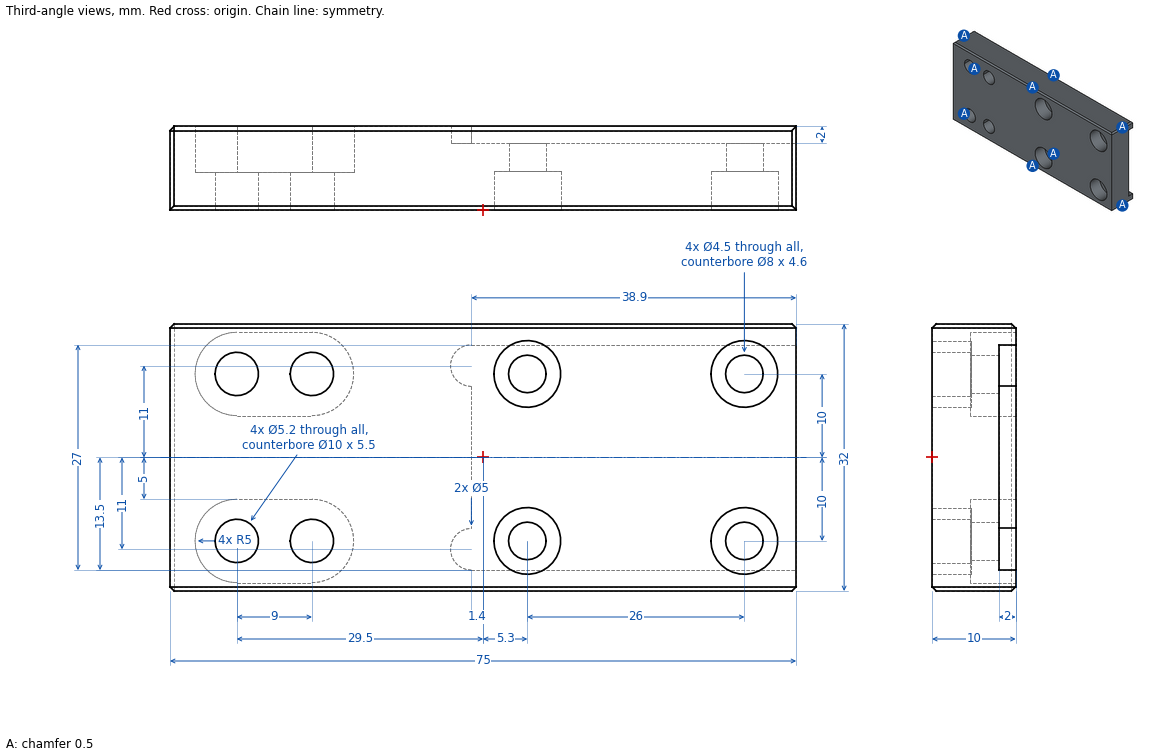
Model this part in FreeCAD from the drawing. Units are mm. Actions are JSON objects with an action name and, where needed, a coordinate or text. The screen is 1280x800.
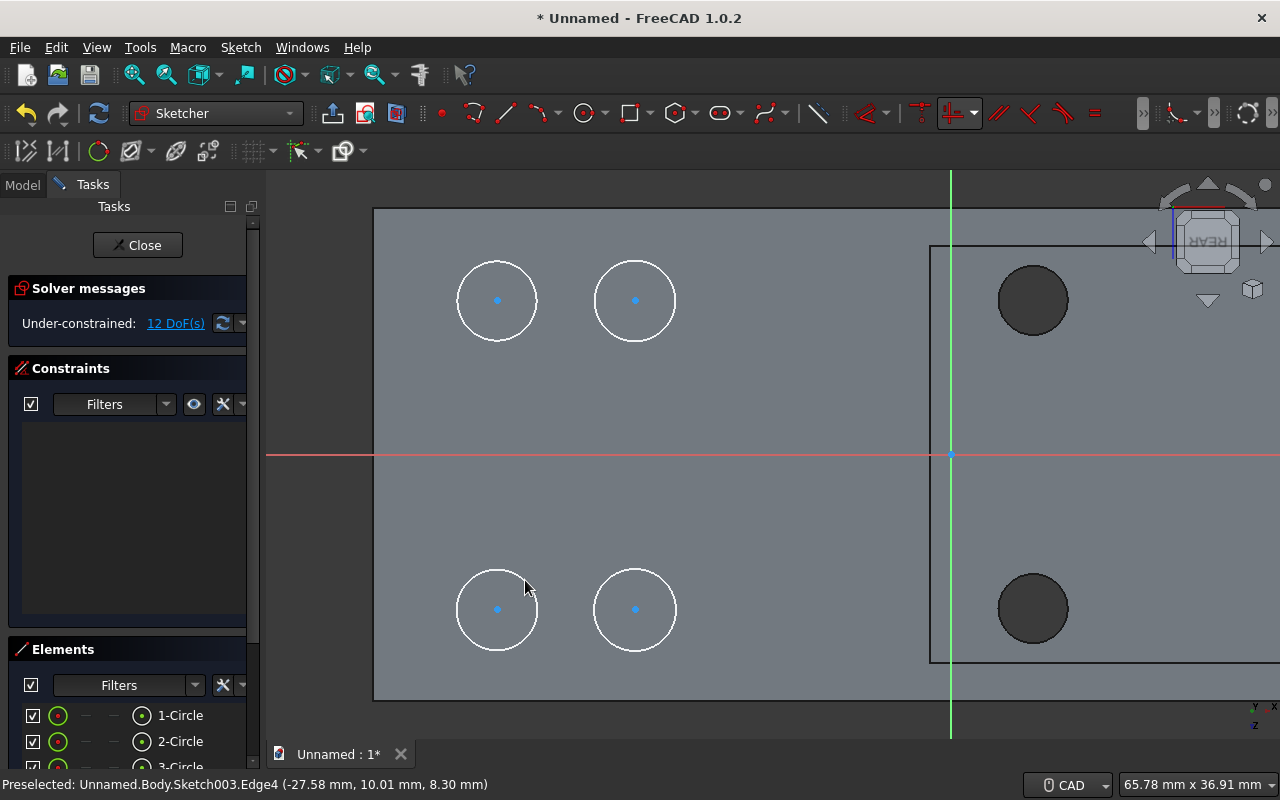
{"action": "left_click", "coordinate": [525, 273]}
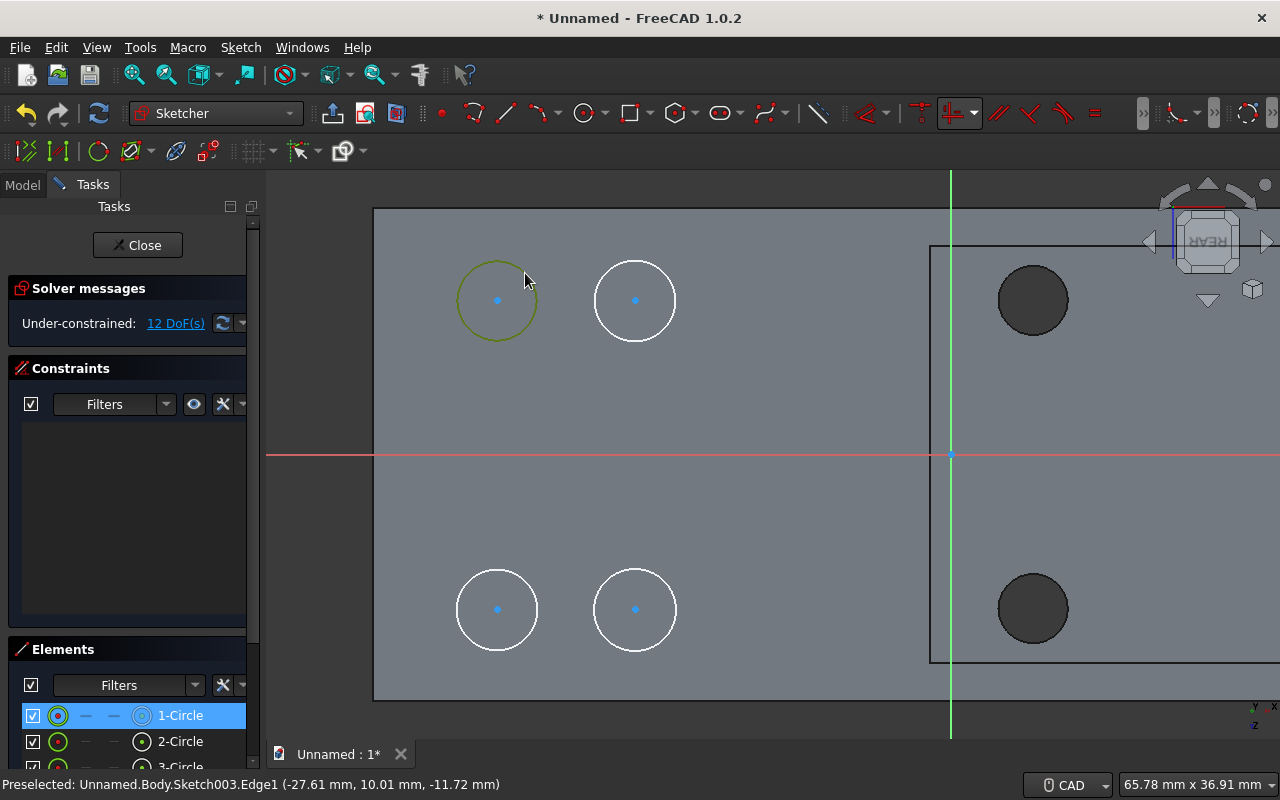
{"action": "left_click", "coordinate": [663, 272]}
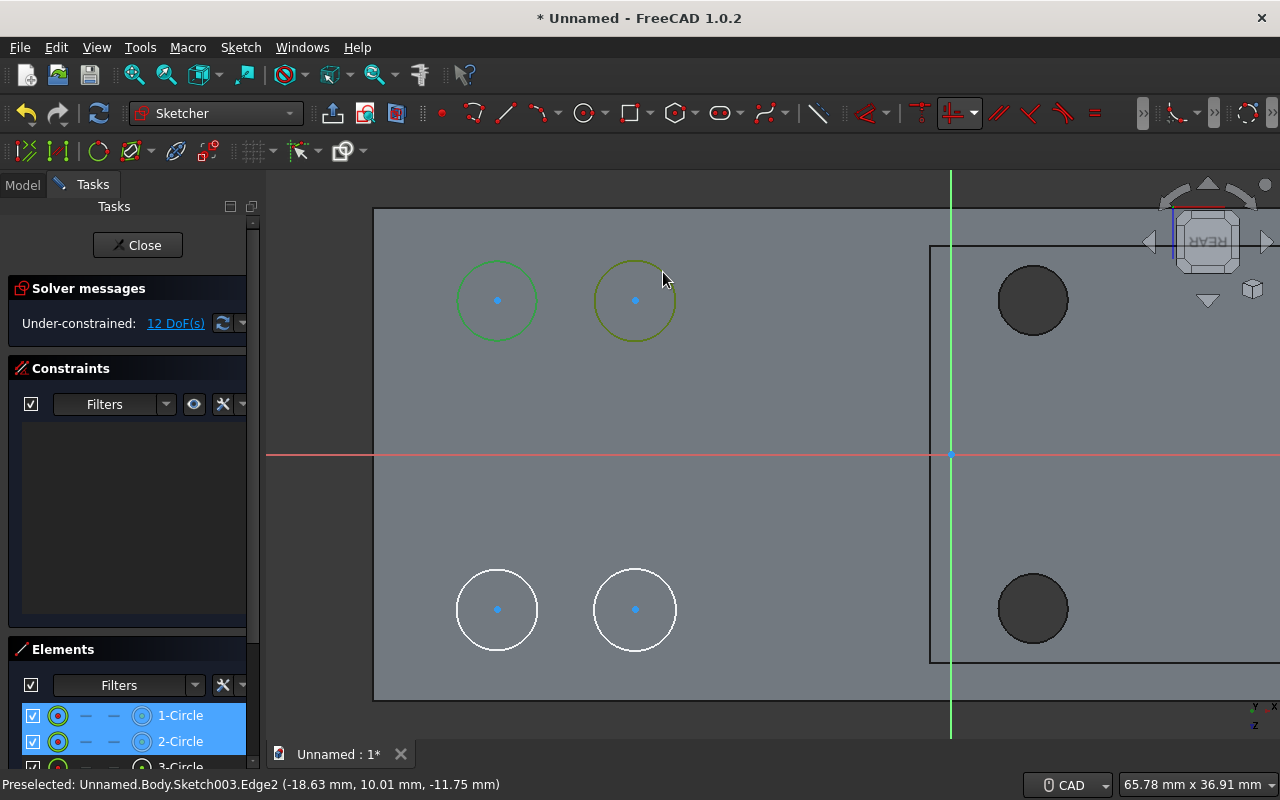
{"action": "left_click", "coordinate": [664, 581]}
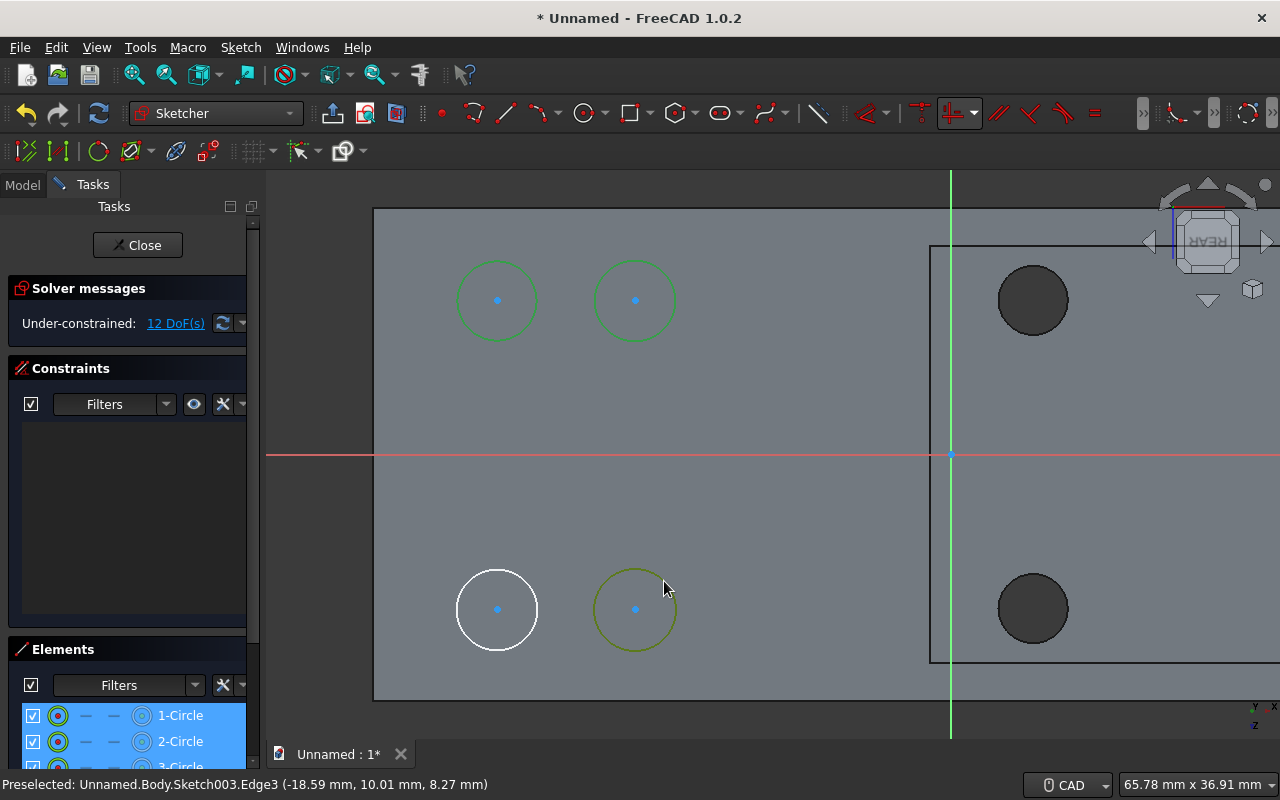
{"action": "left_click", "coordinate": [525, 581]}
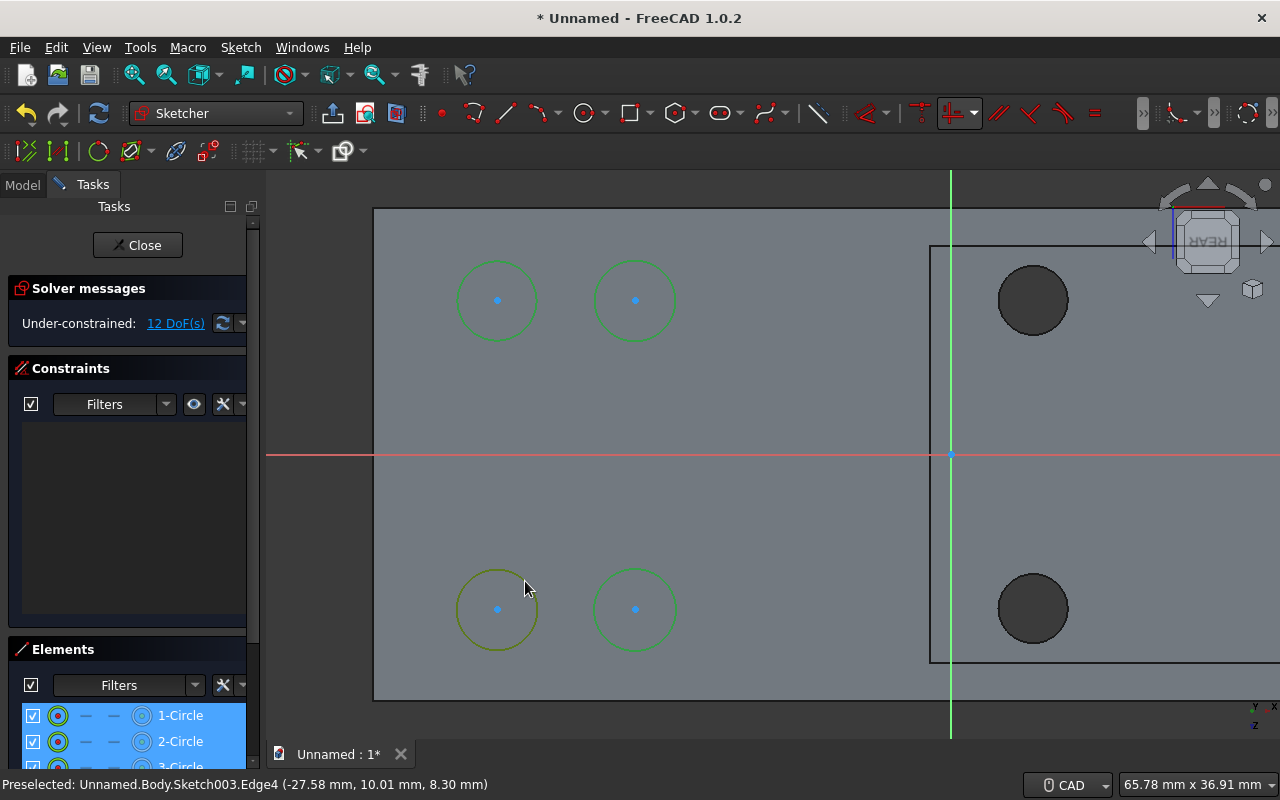
{"action": "left_click", "coordinate": [1096, 114]}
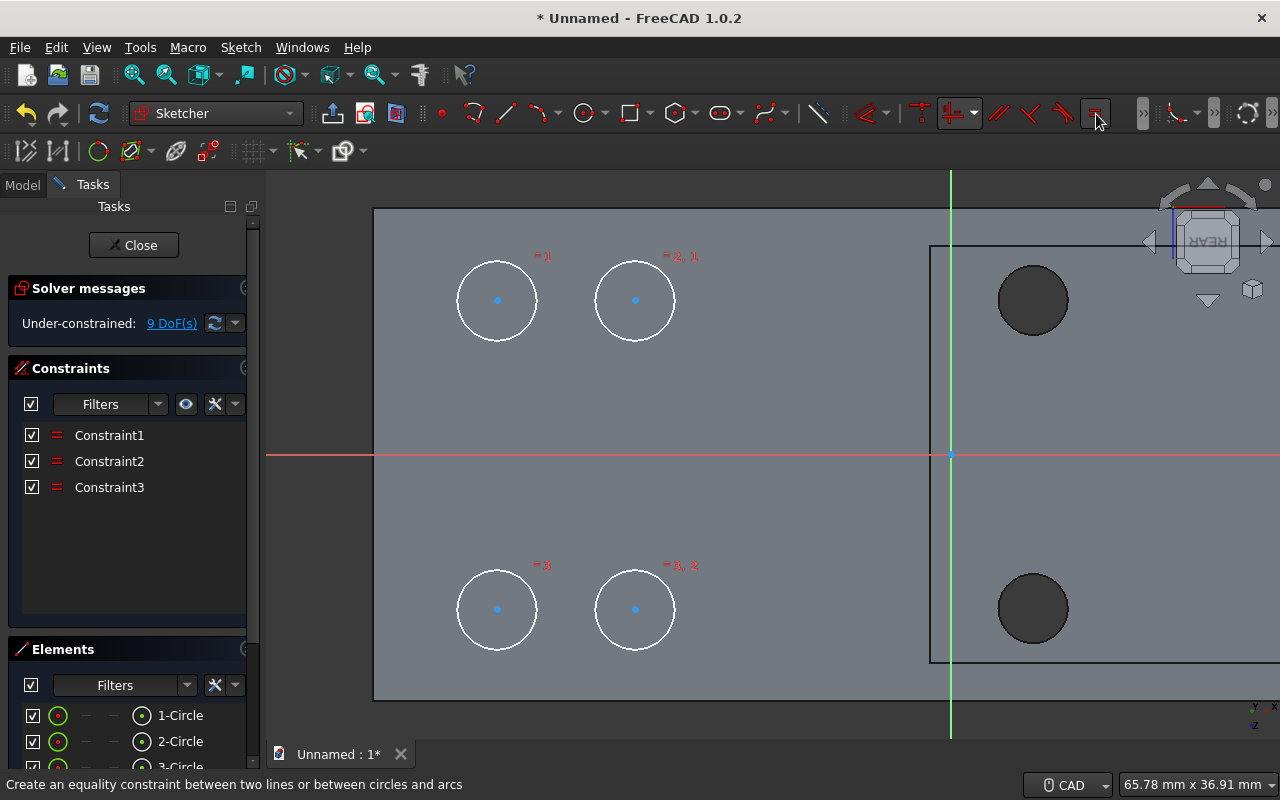
{"action": "left_click", "coordinate": [497, 301]}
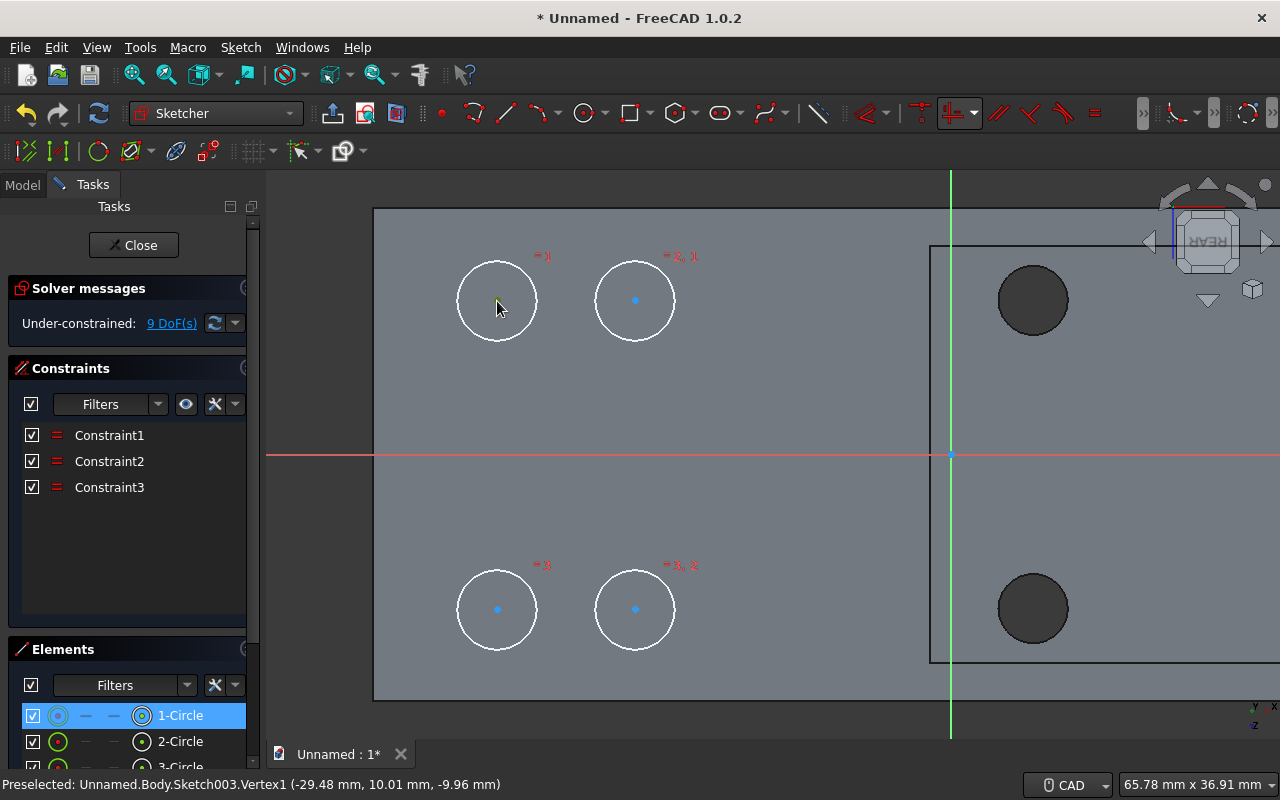
{"action": "left_click", "coordinate": [635, 301]}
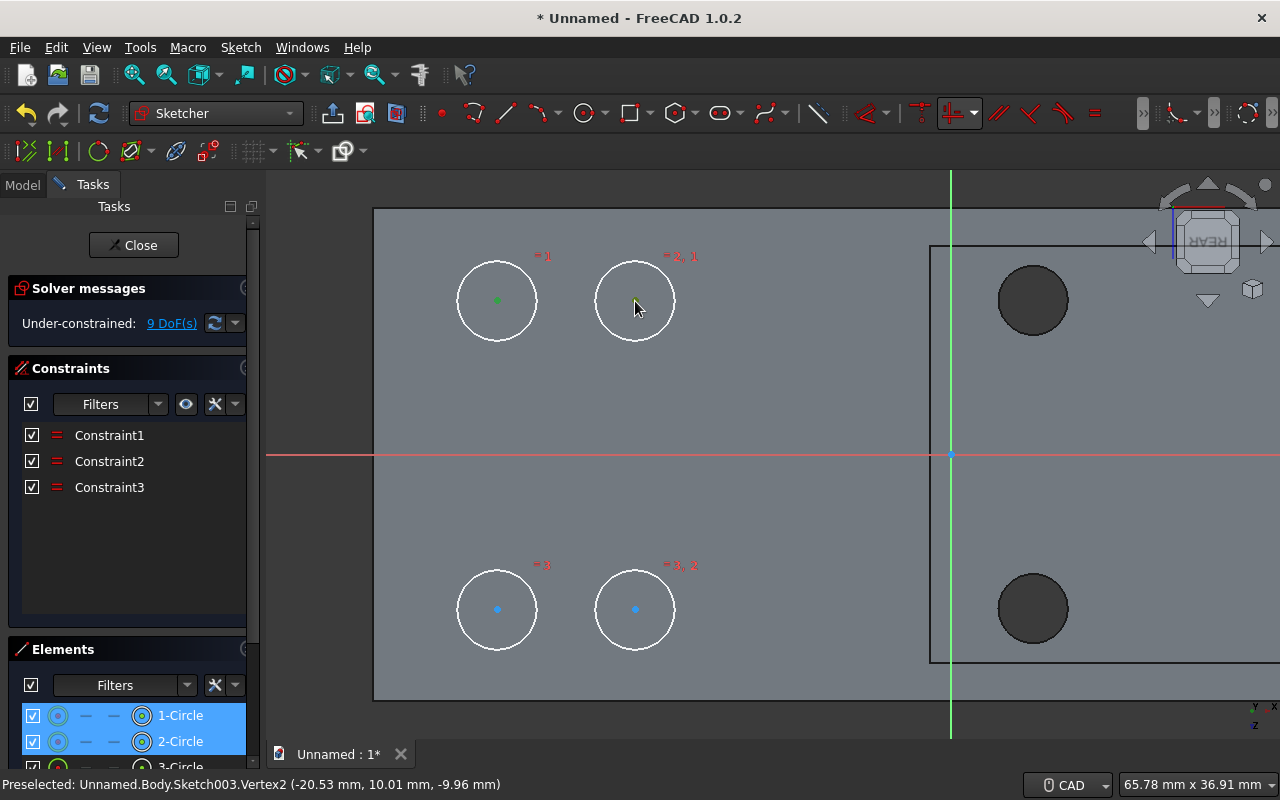
{"action": "left_click", "coordinate": [976, 114]}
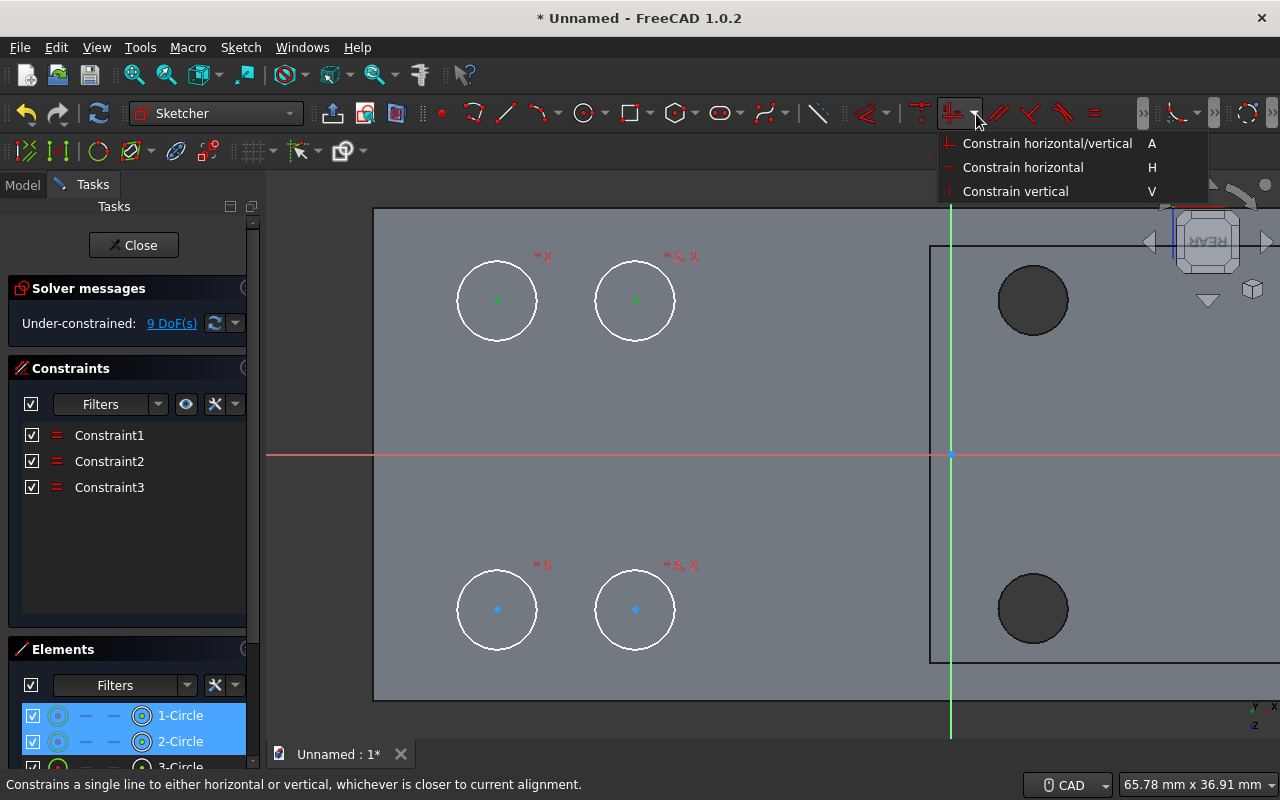
{"action": "left_click", "coordinate": [1073, 167]}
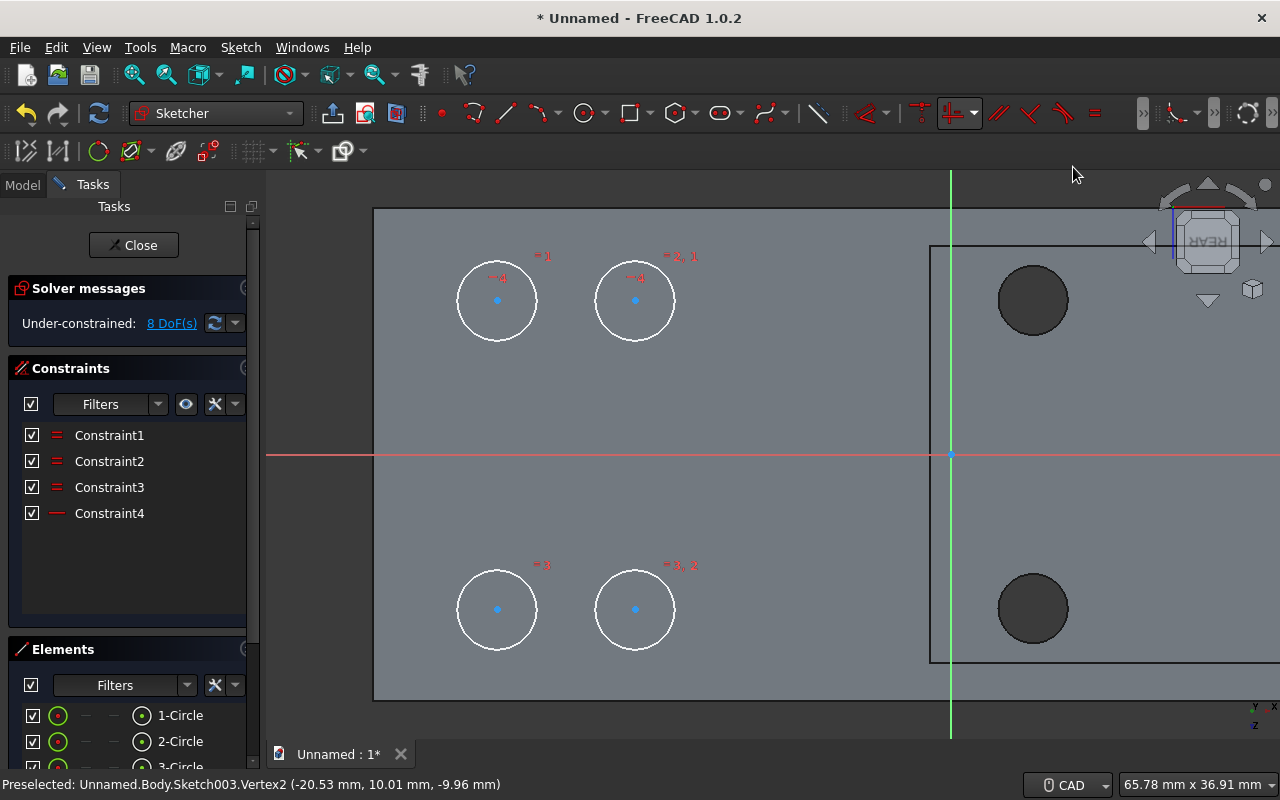
{"action": "left_click", "coordinate": [635, 301]}